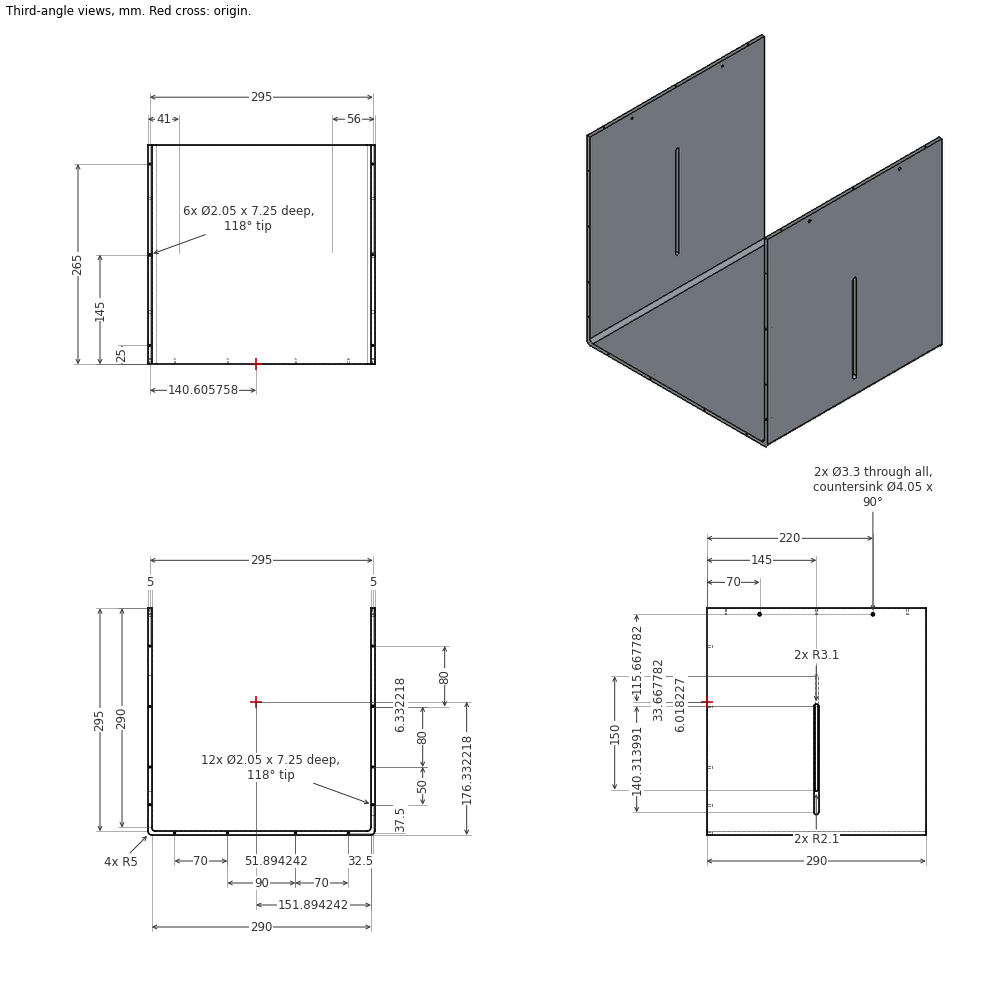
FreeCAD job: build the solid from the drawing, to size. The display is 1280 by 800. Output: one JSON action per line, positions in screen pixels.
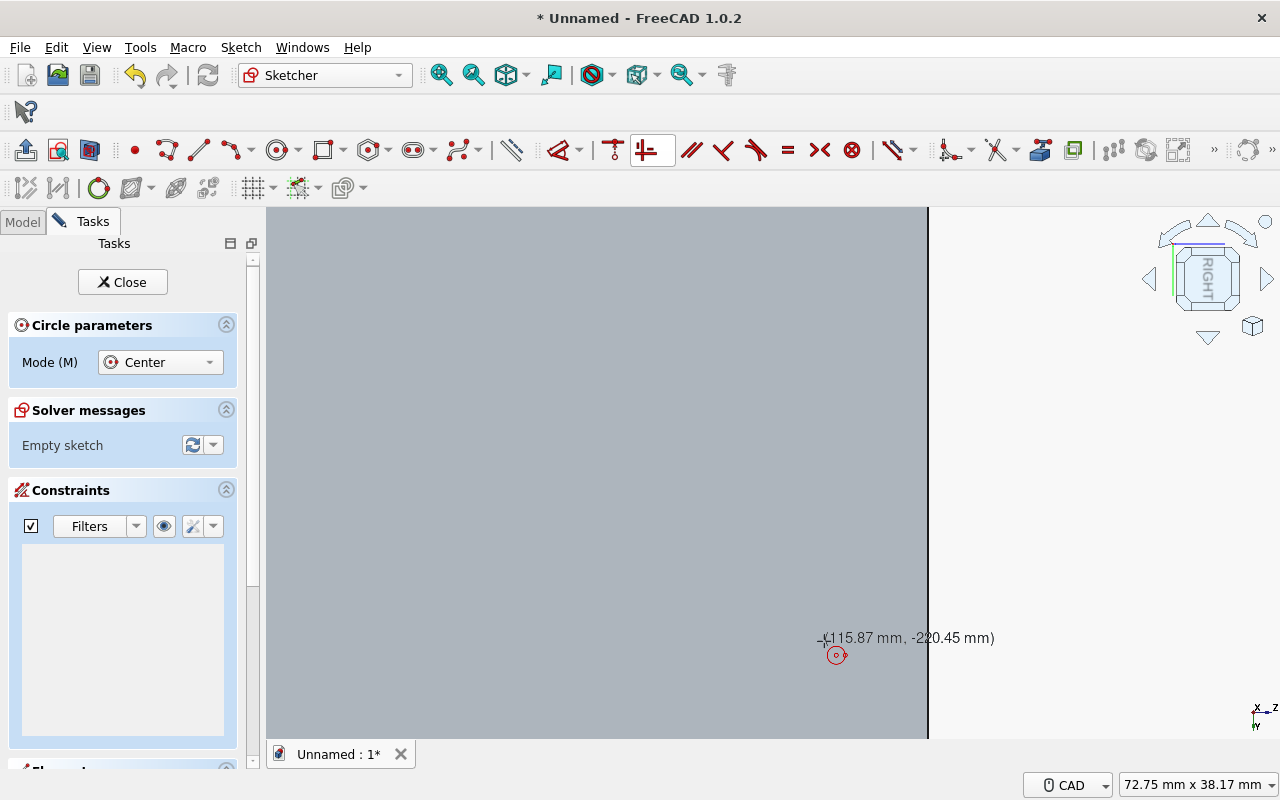
{"action": "scroll", "coordinate": [790, 642], "scroll_direction": "down", "scroll_amount": 11}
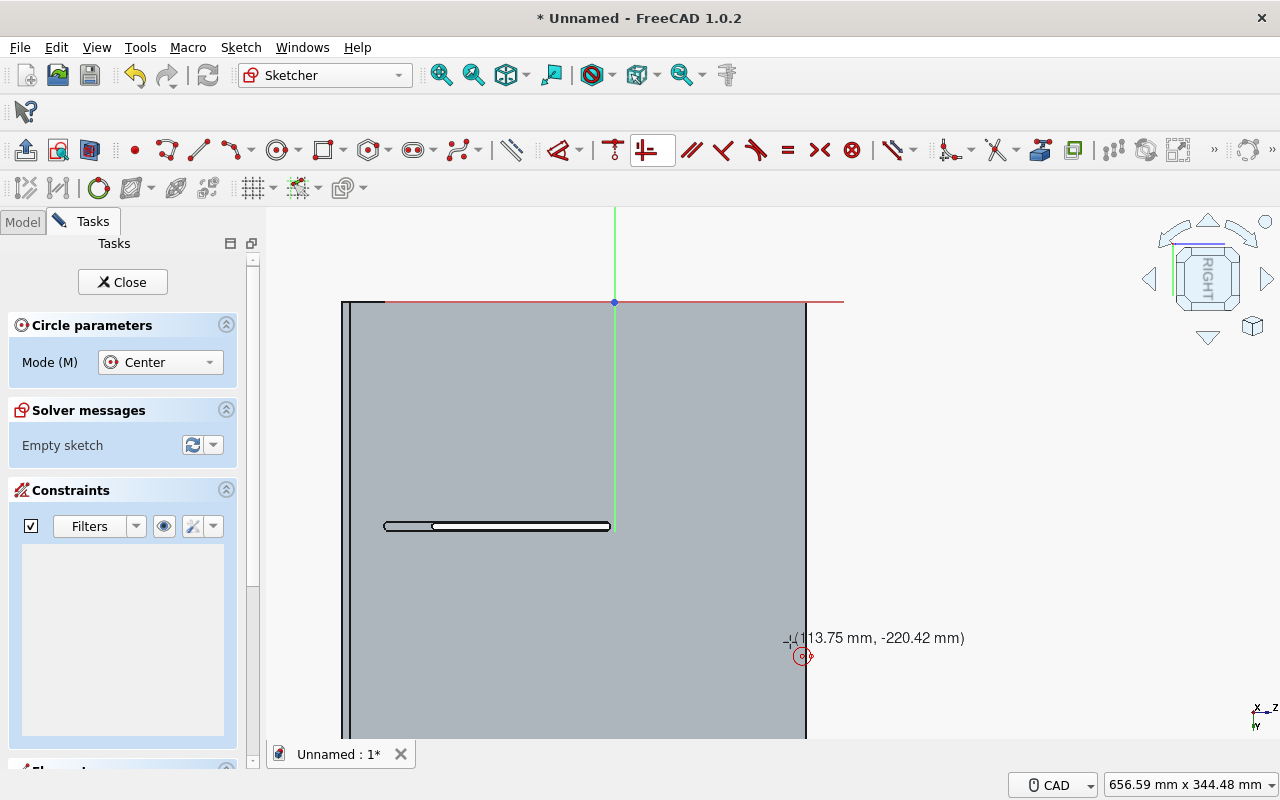
{"action": "left_click", "coordinate": [793, 642]}
{"action": "mouse_move", "coordinate": [795, 640]}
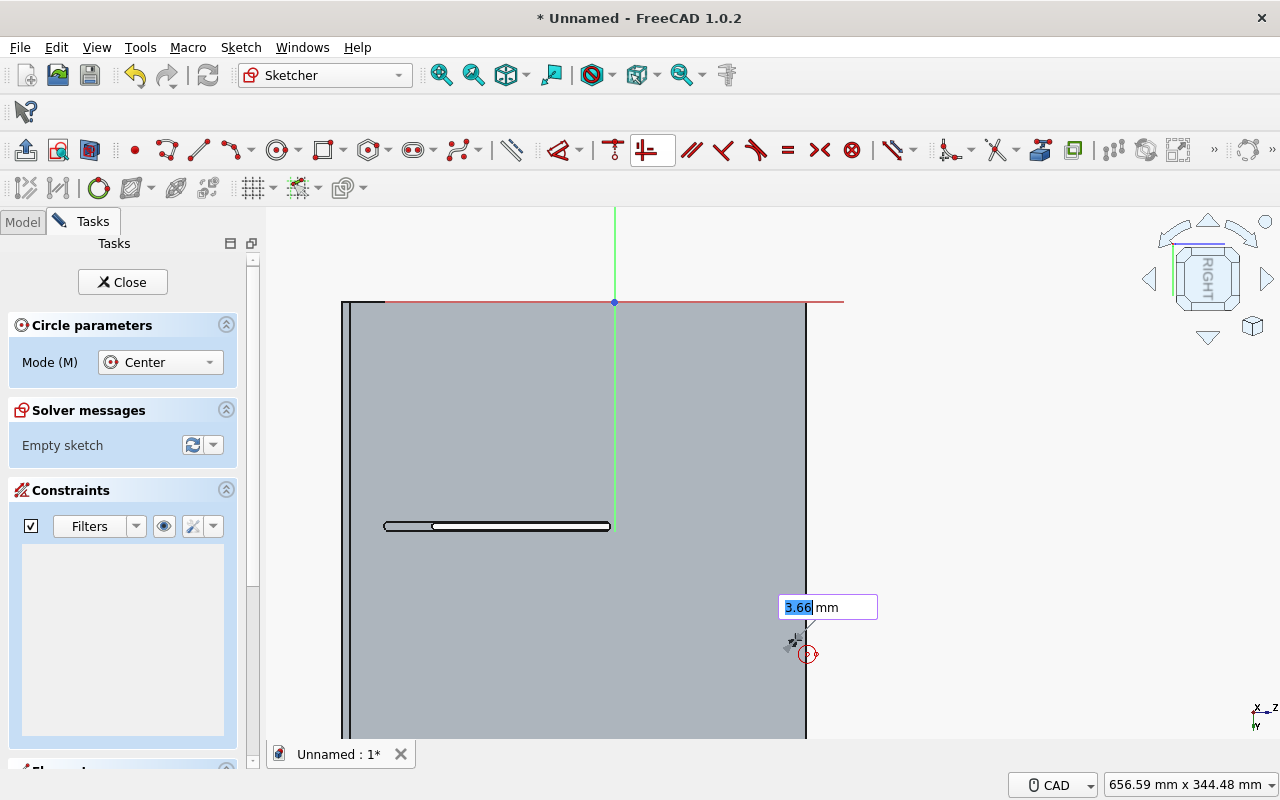
{"action": "type", "text": "3.3"}
{"action": "key", "text": "Return"}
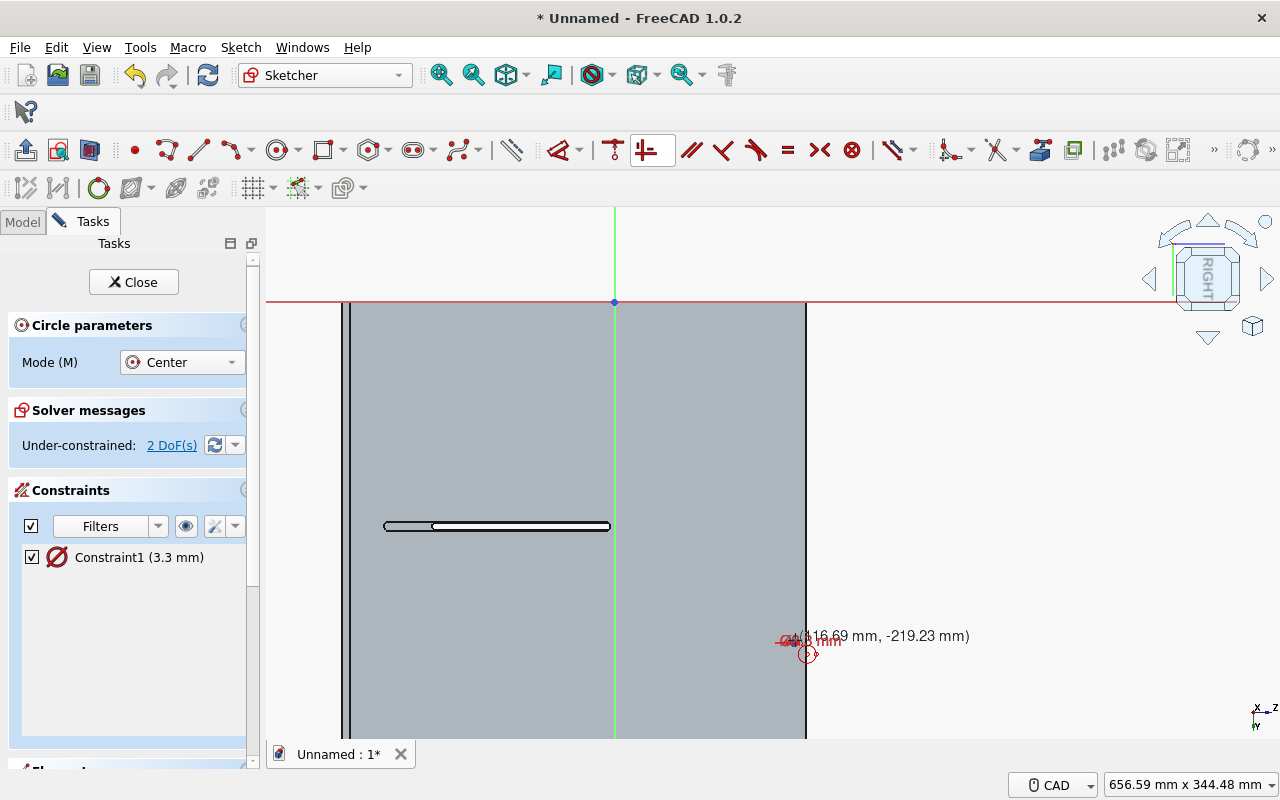
{"action": "scroll", "coordinate": [793, 411], "scroll_direction": "up", "scroll_amount": 11}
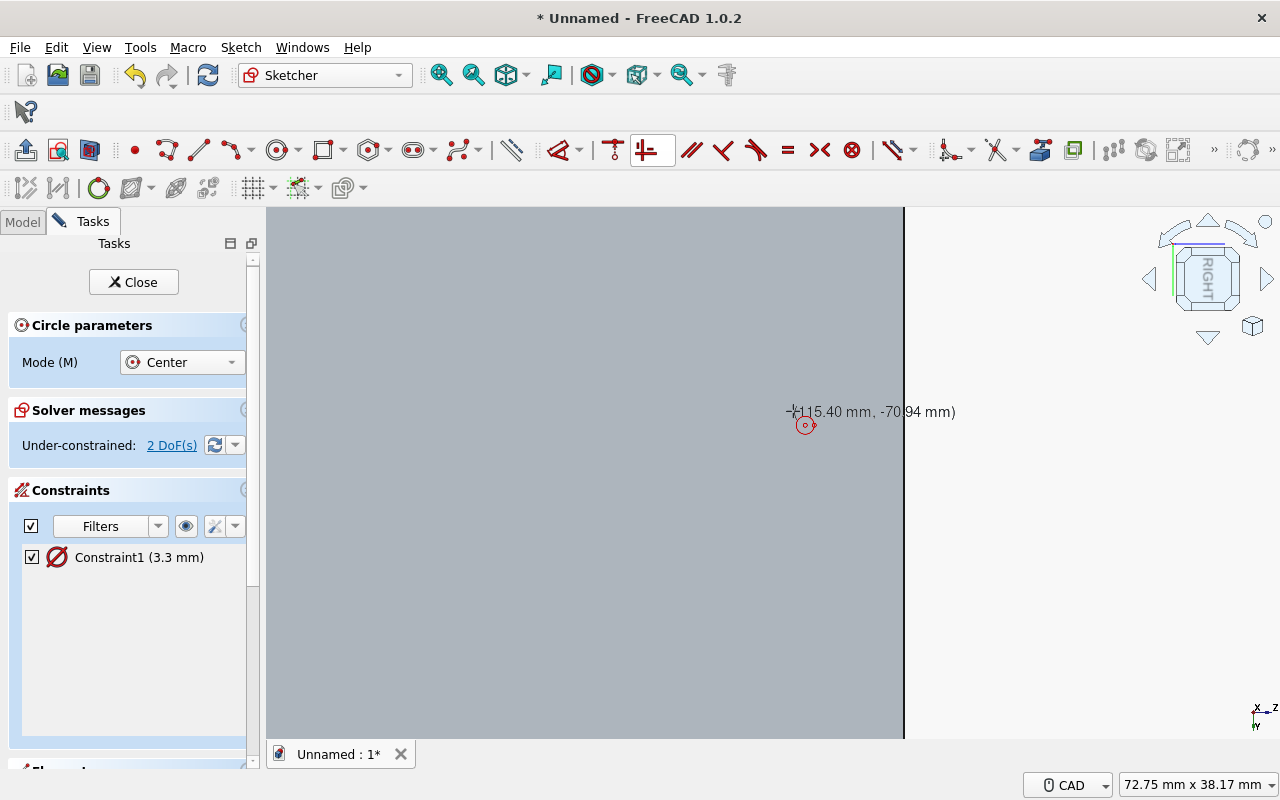
{"action": "scroll", "coordinate": [793, 411], "scroll_direction": "down", "scroll_amount": 11}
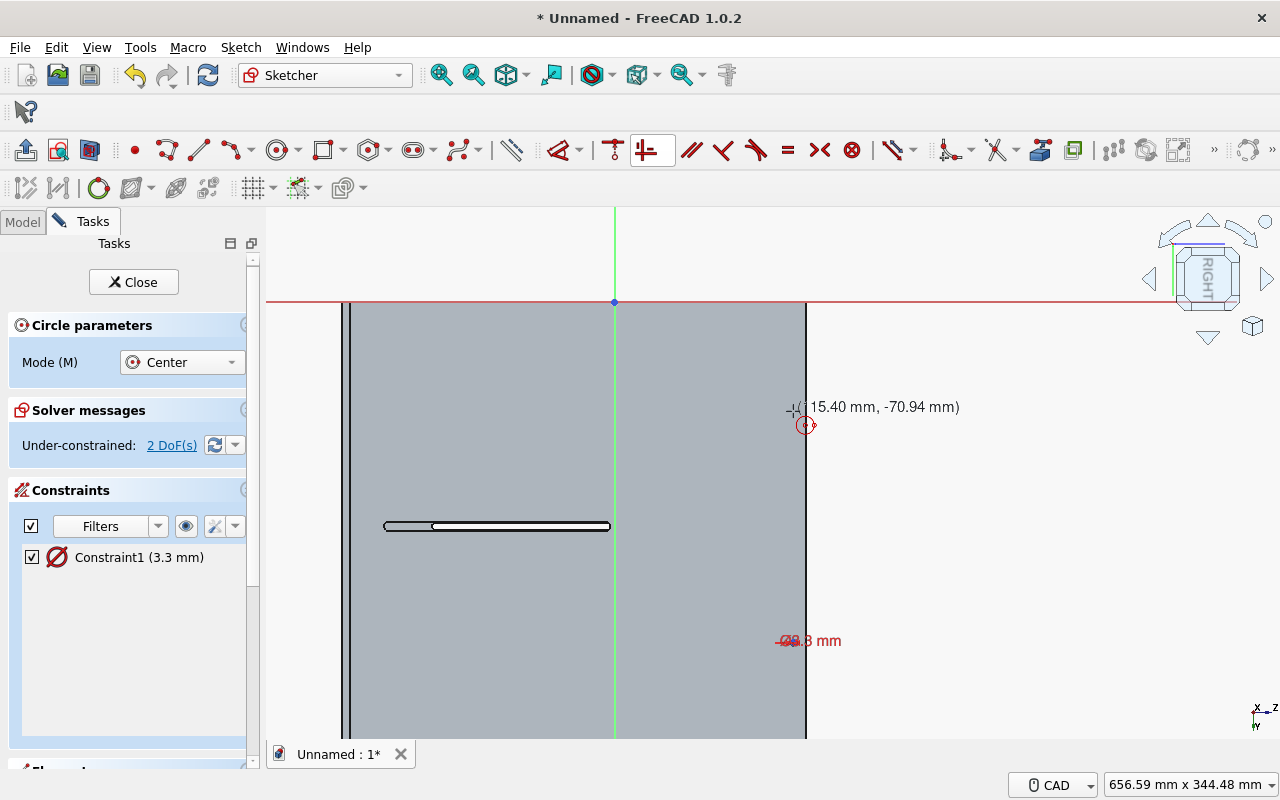
{"action": "left_click", "coordinate": [793, 411]}
{"action": "mouse_move", "coordinate": [795, 409]}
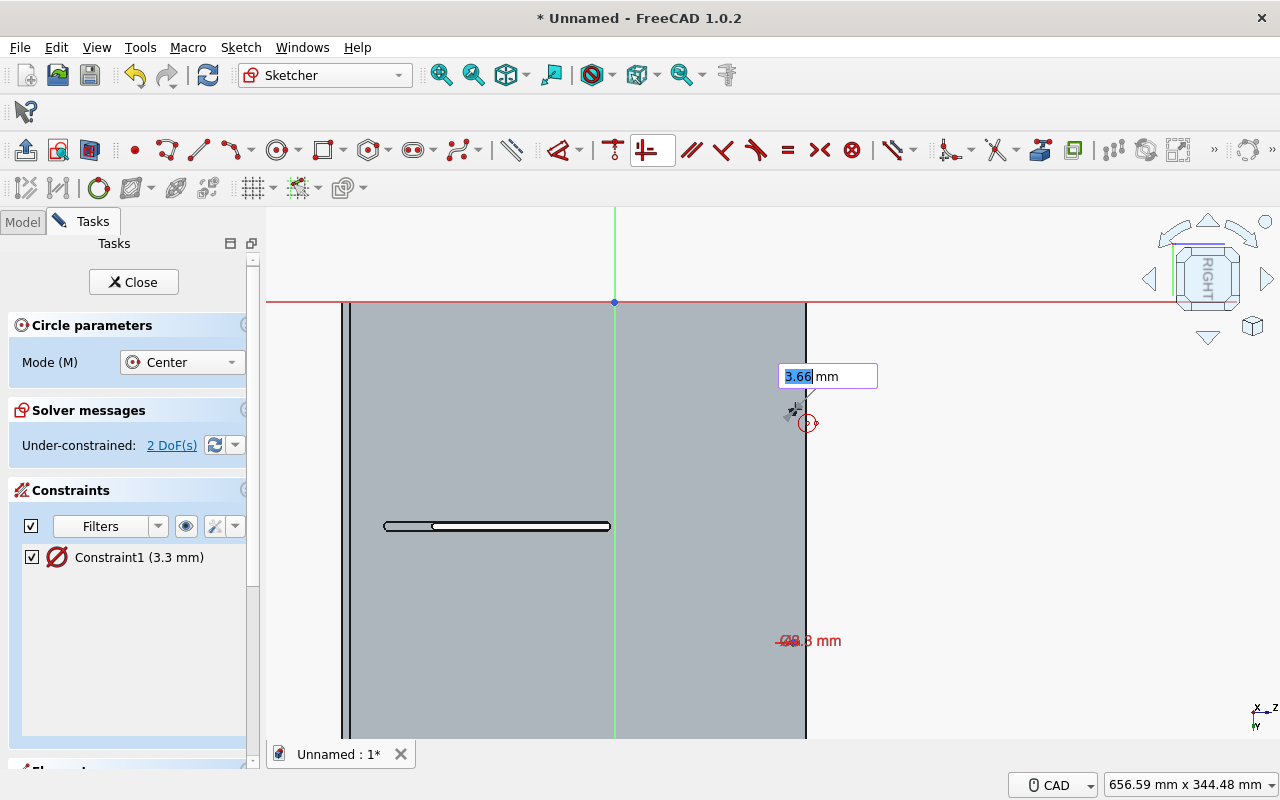
{"action": "type", "text": "3.3"}
{"action": "key", "text": "Return"}
{"action": "key", "text": "Escape"}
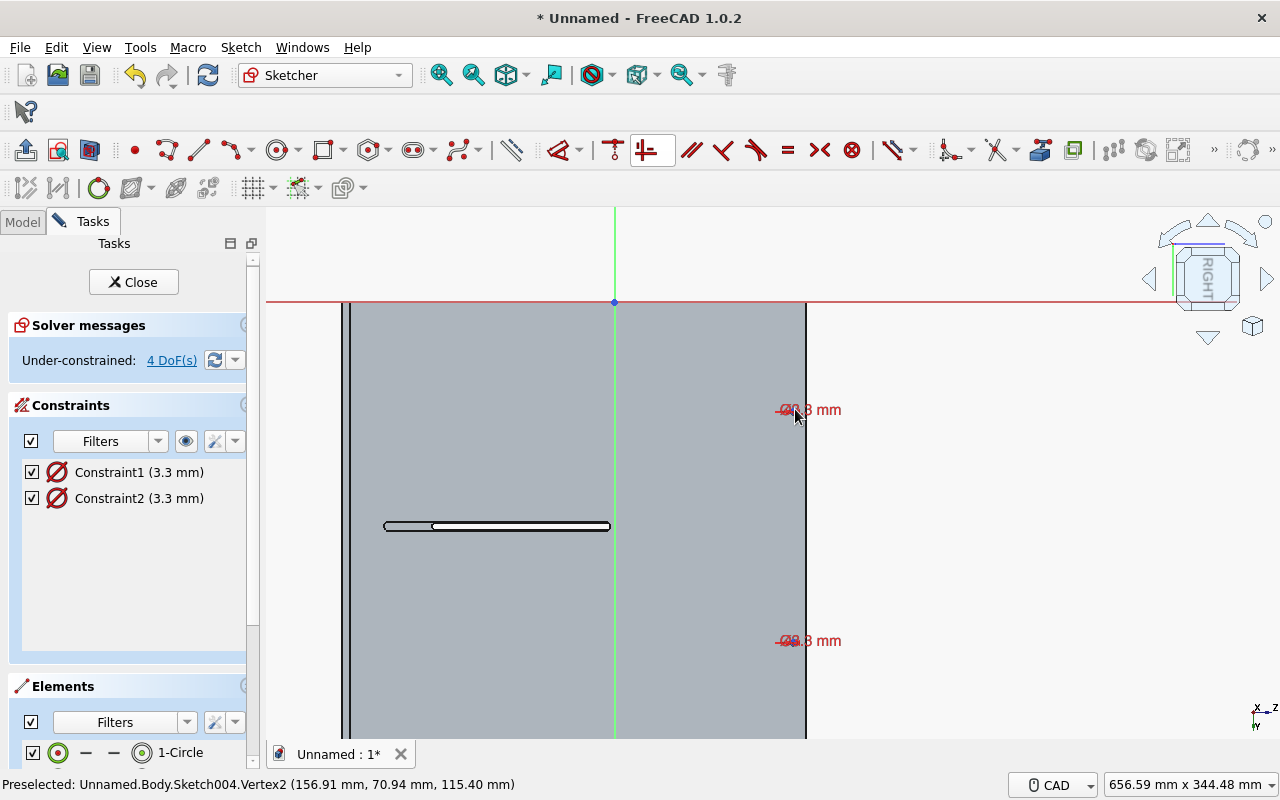
{"action": "left_click", "coordinate": [793, 643]}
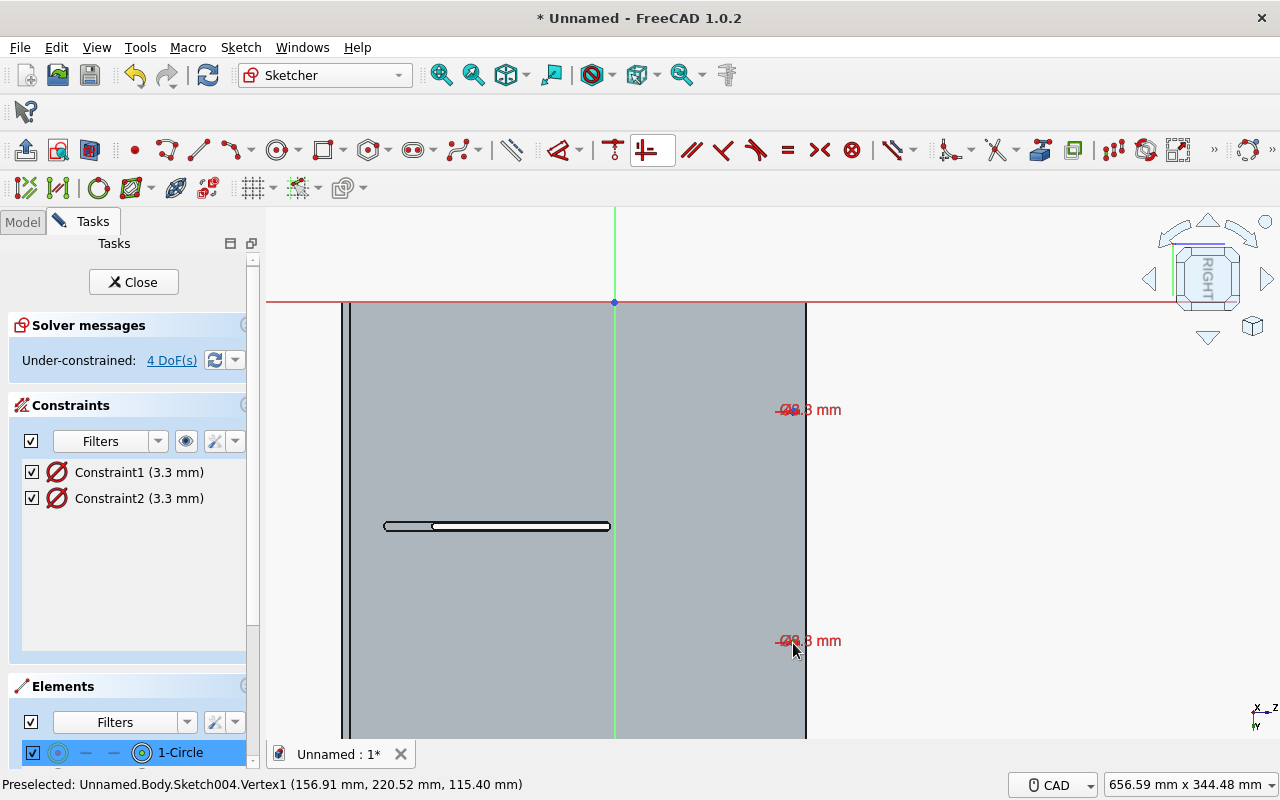
{"action": "left_click", "coordinate": [793, 412]}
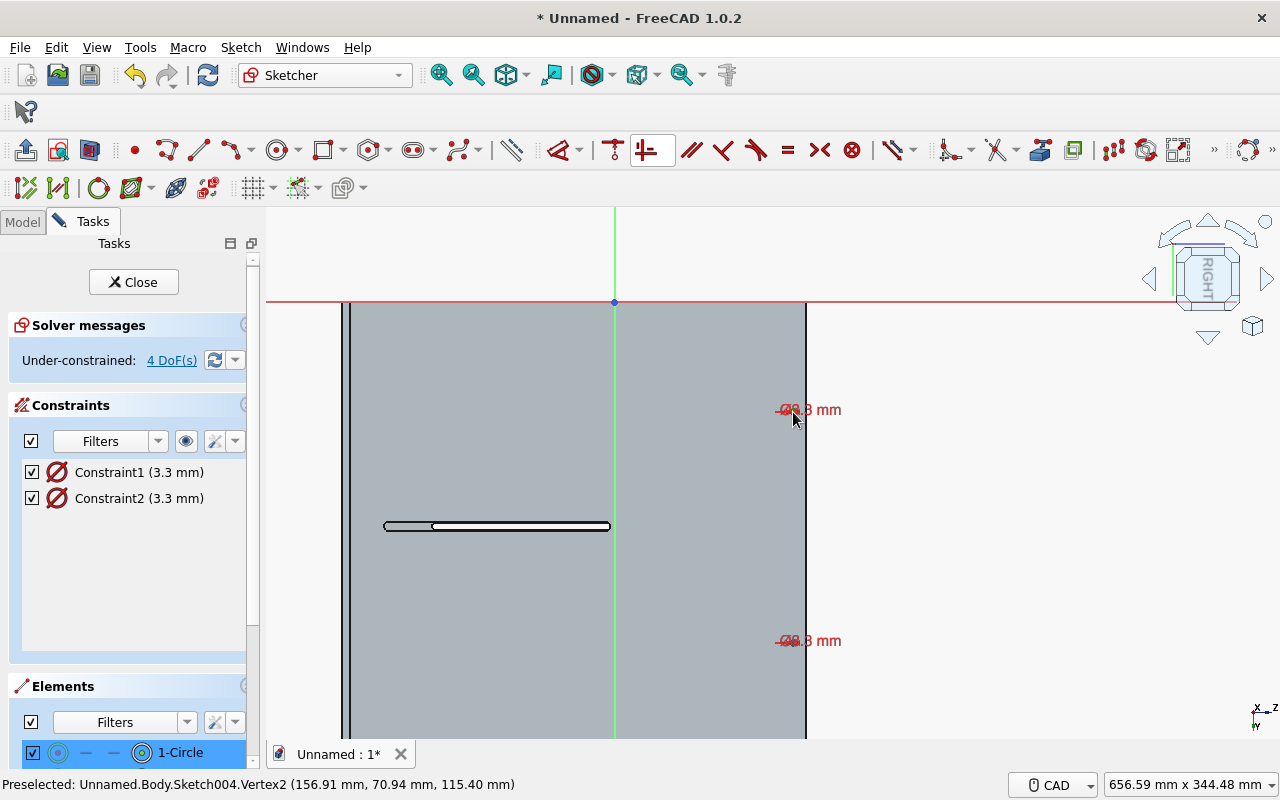
{"action": "left_click", "coordinate": [670, 150]}